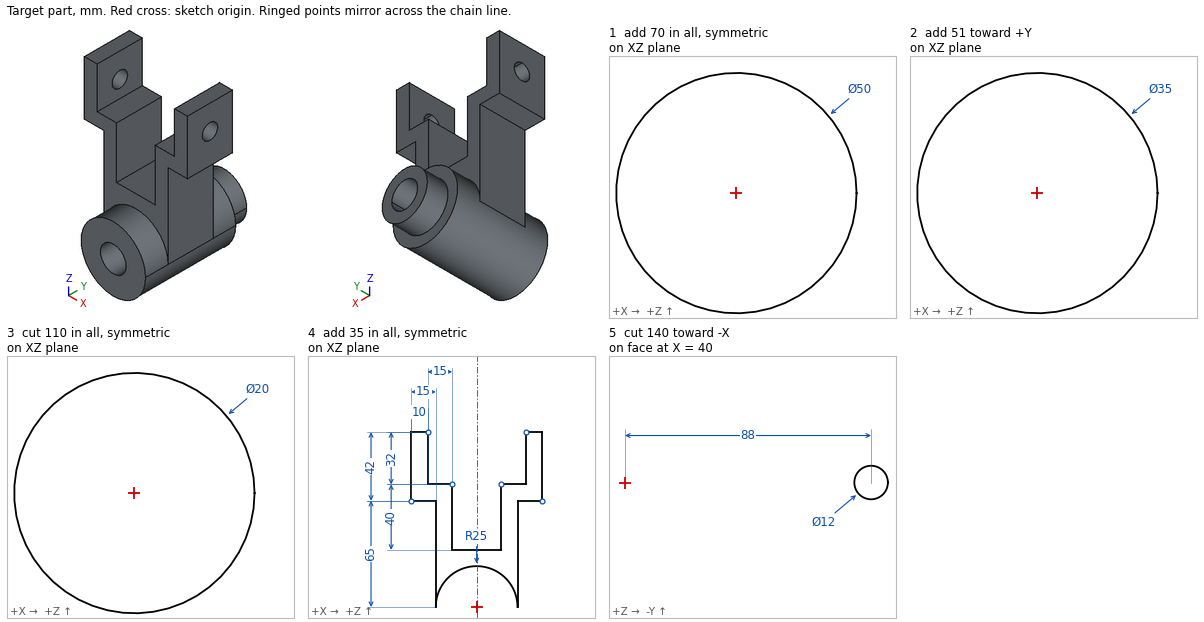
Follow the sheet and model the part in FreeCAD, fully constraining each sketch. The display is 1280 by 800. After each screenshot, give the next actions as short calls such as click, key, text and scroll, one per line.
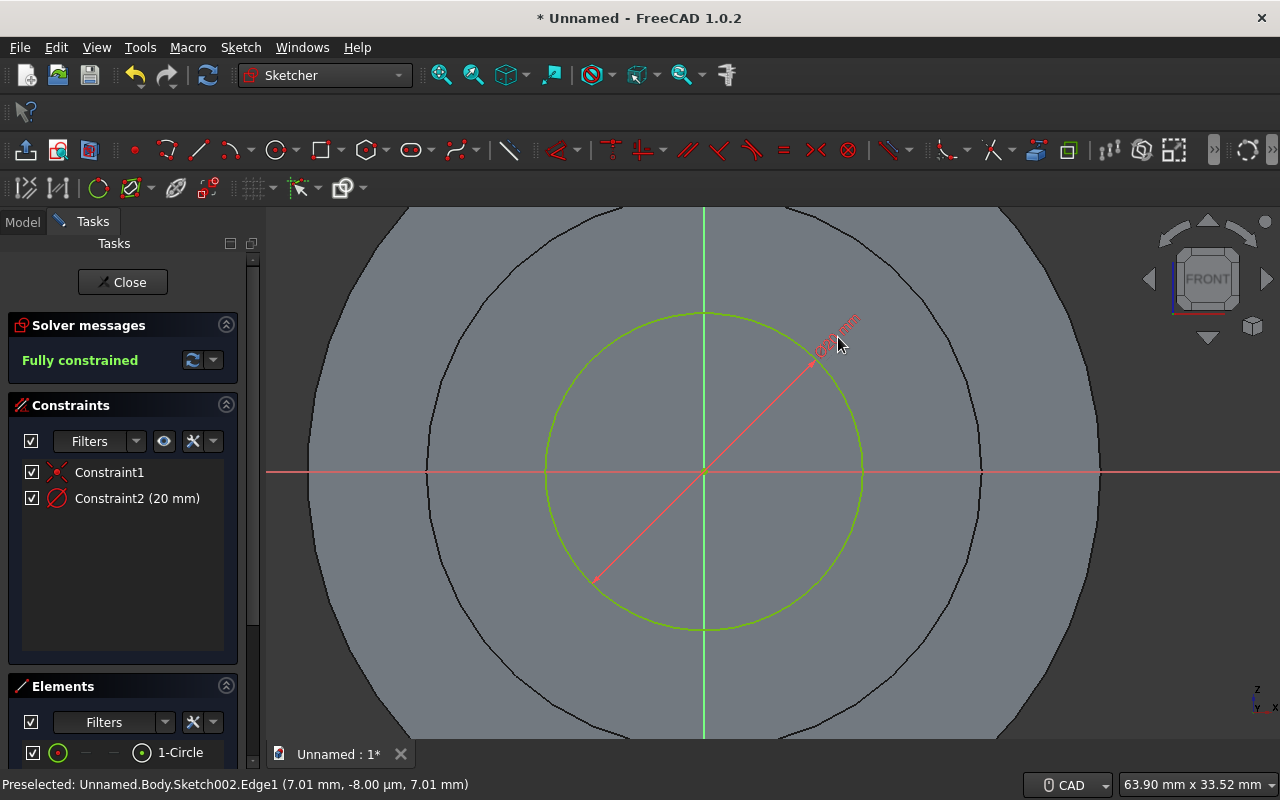
click(123, 282)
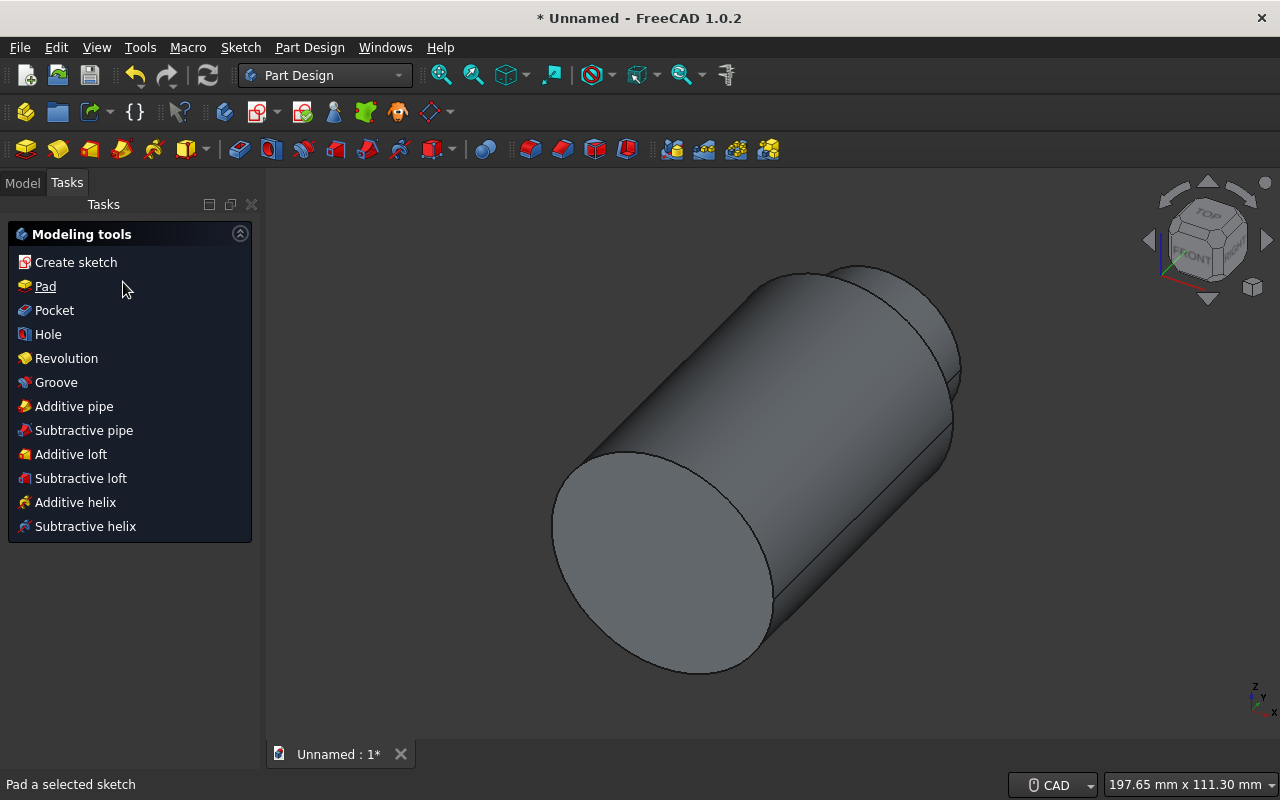
click(240, 150)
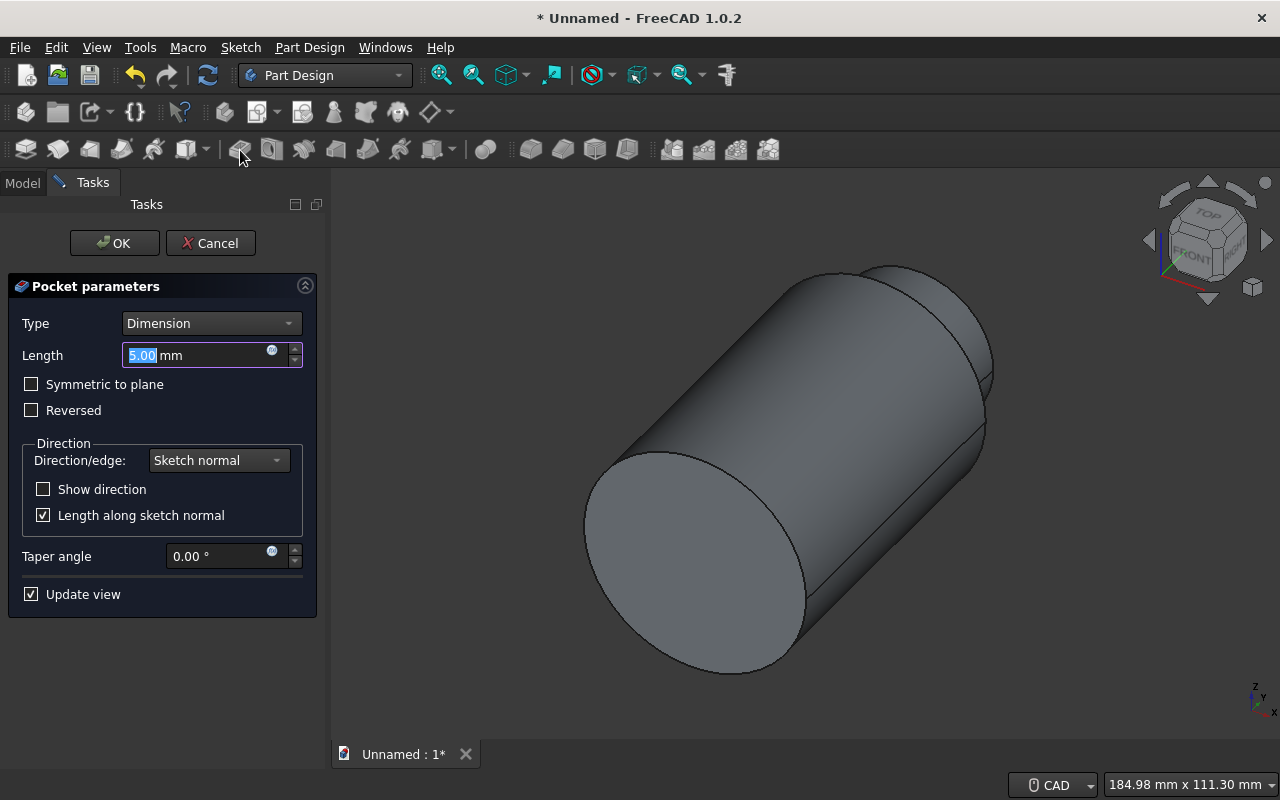
text(110)
key(Tab)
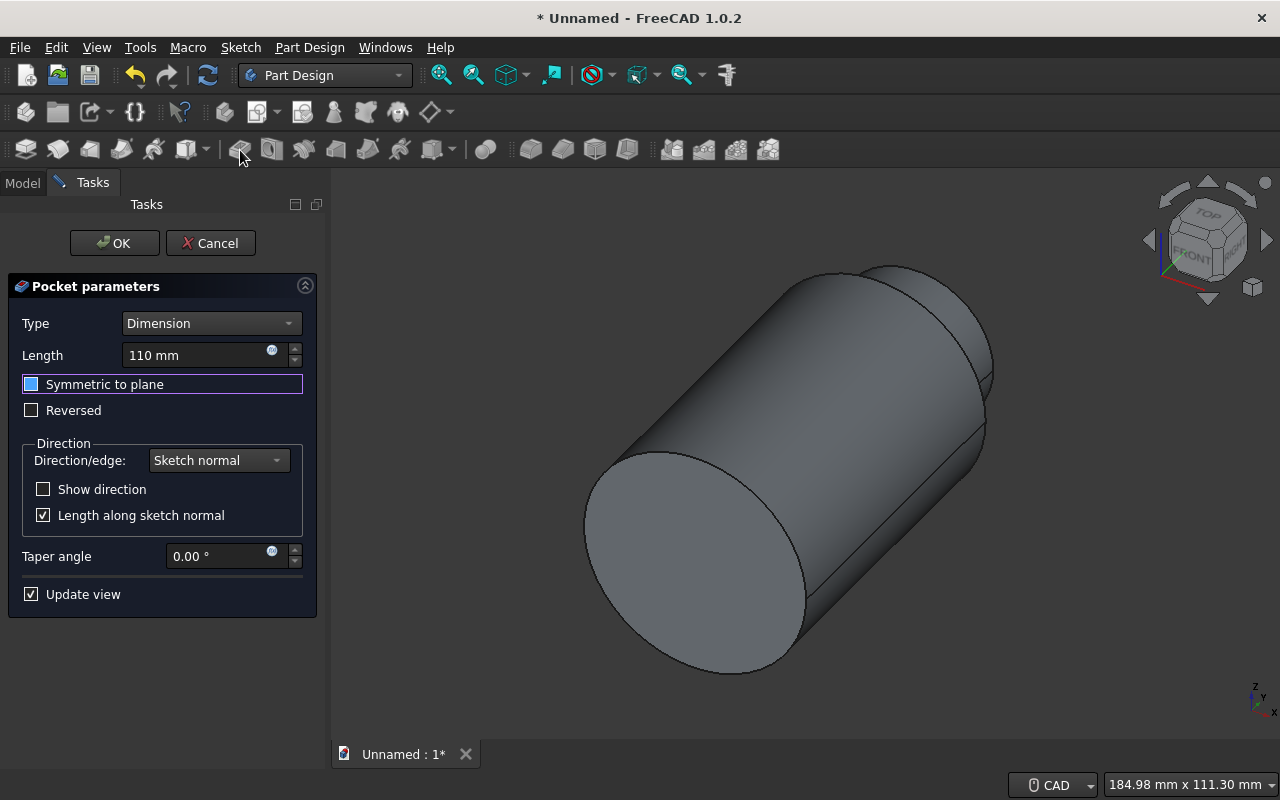
click(30, 384)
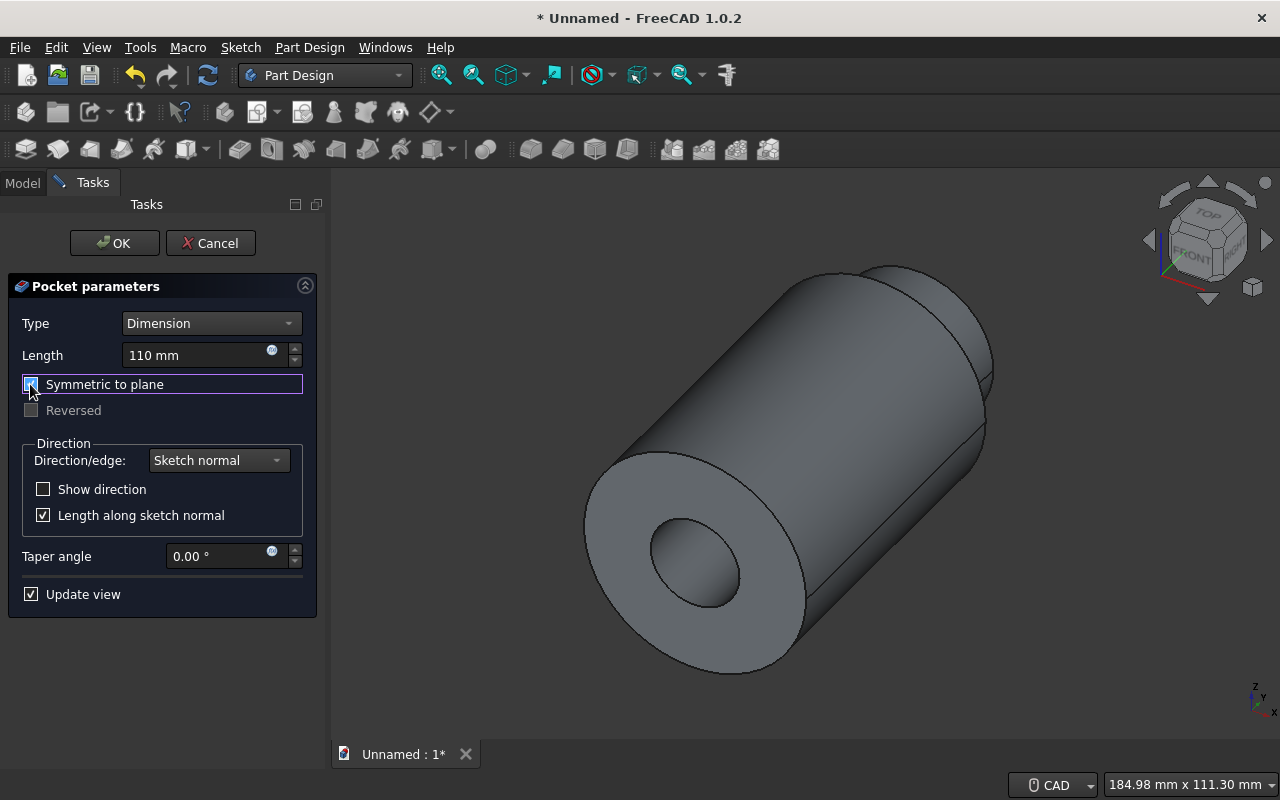
click(115, 243)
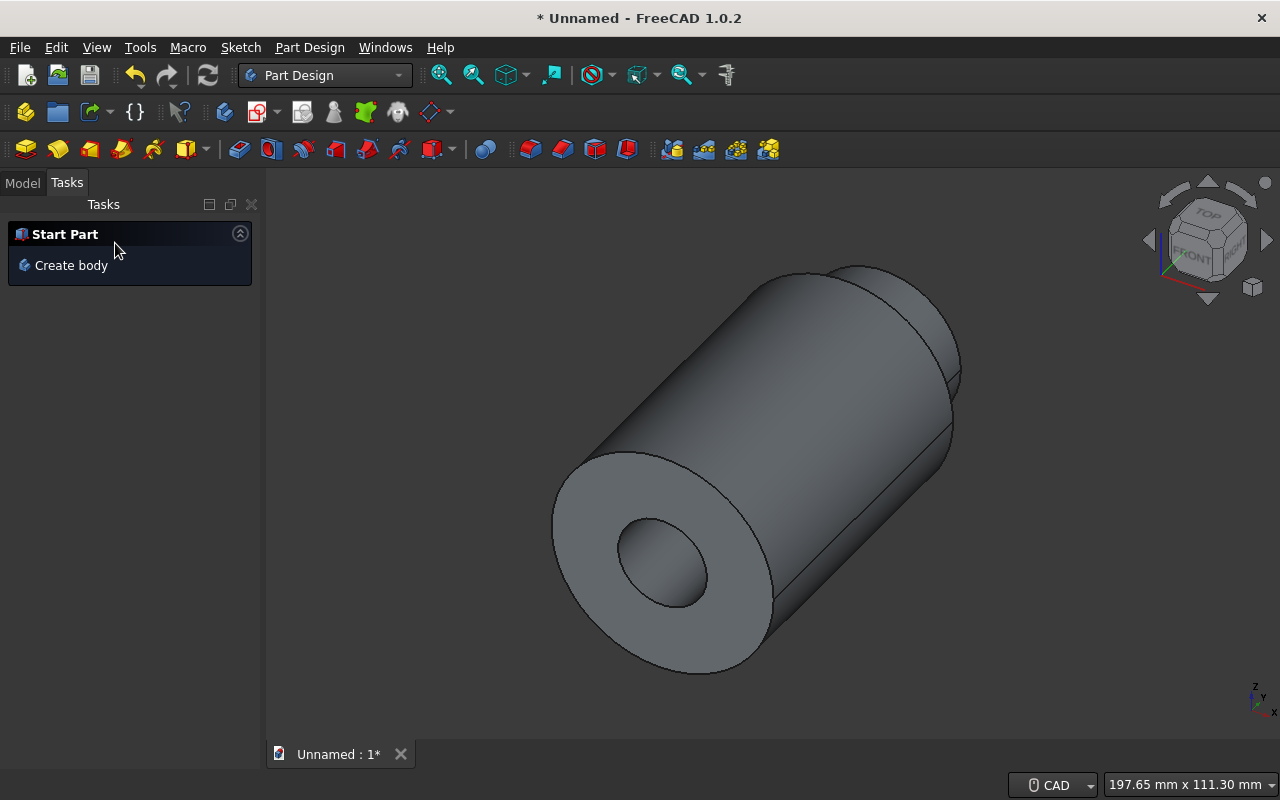
click(258, 112)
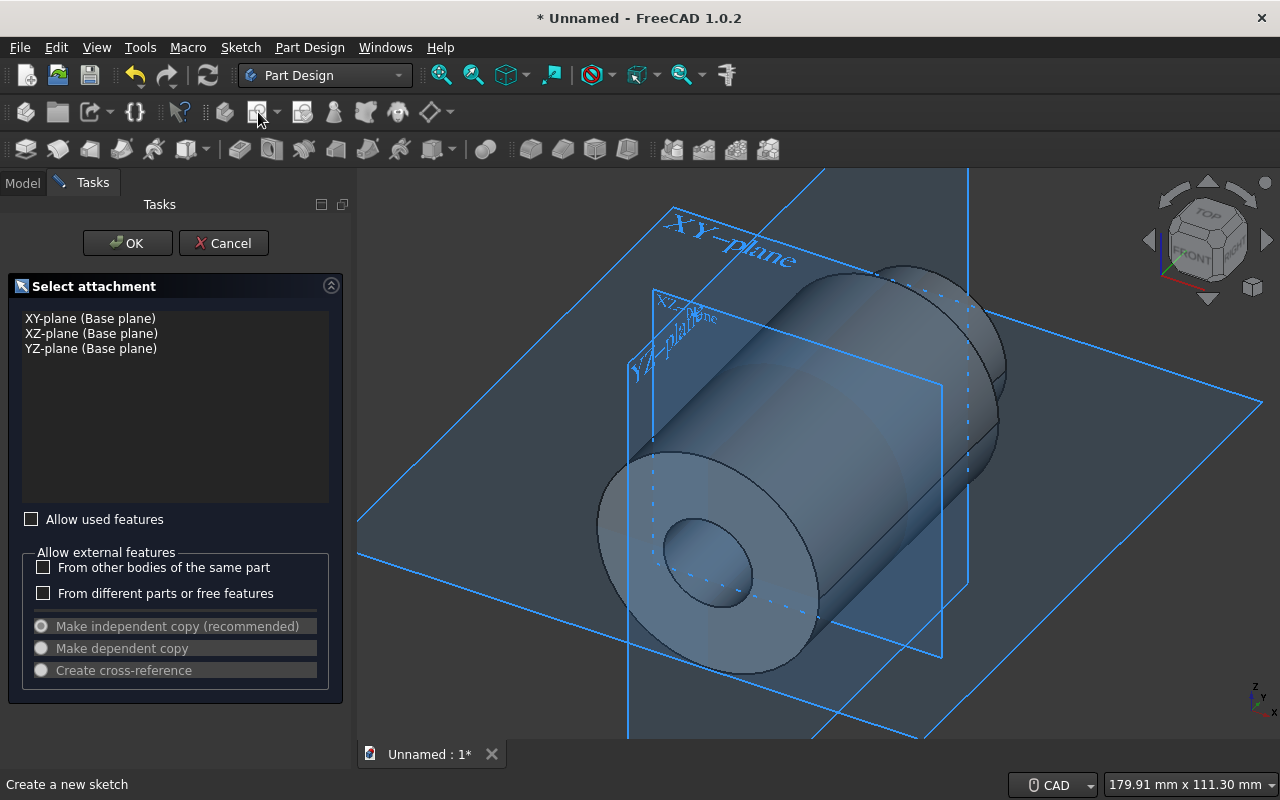
click(82, 334)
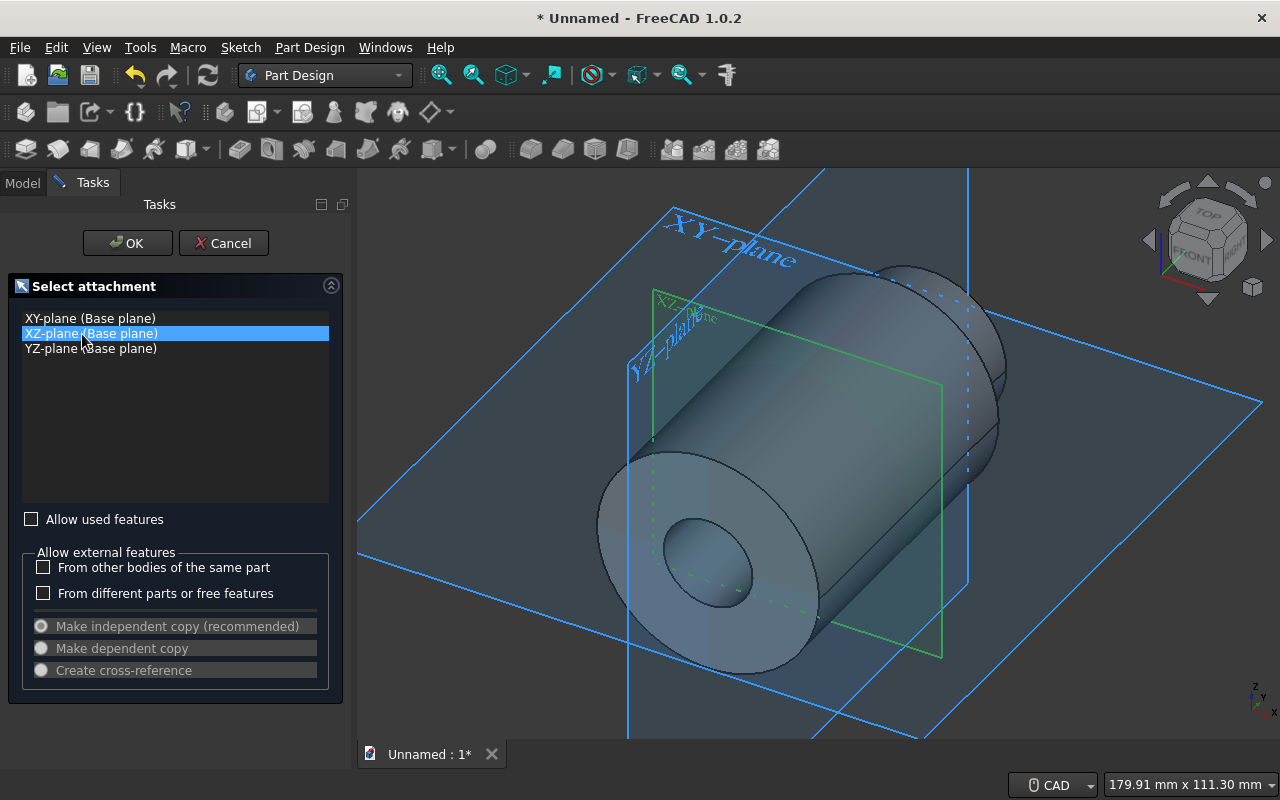
click(128, 243)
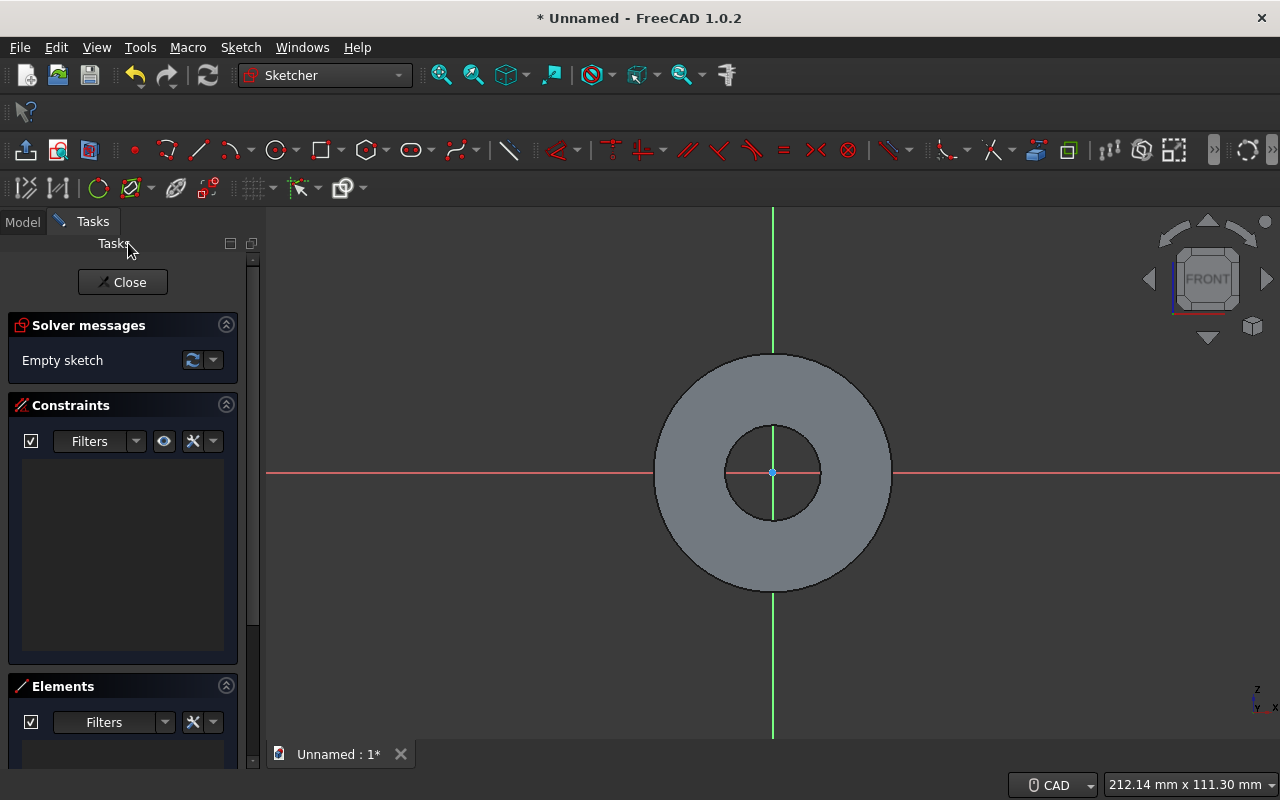
click(90, 150)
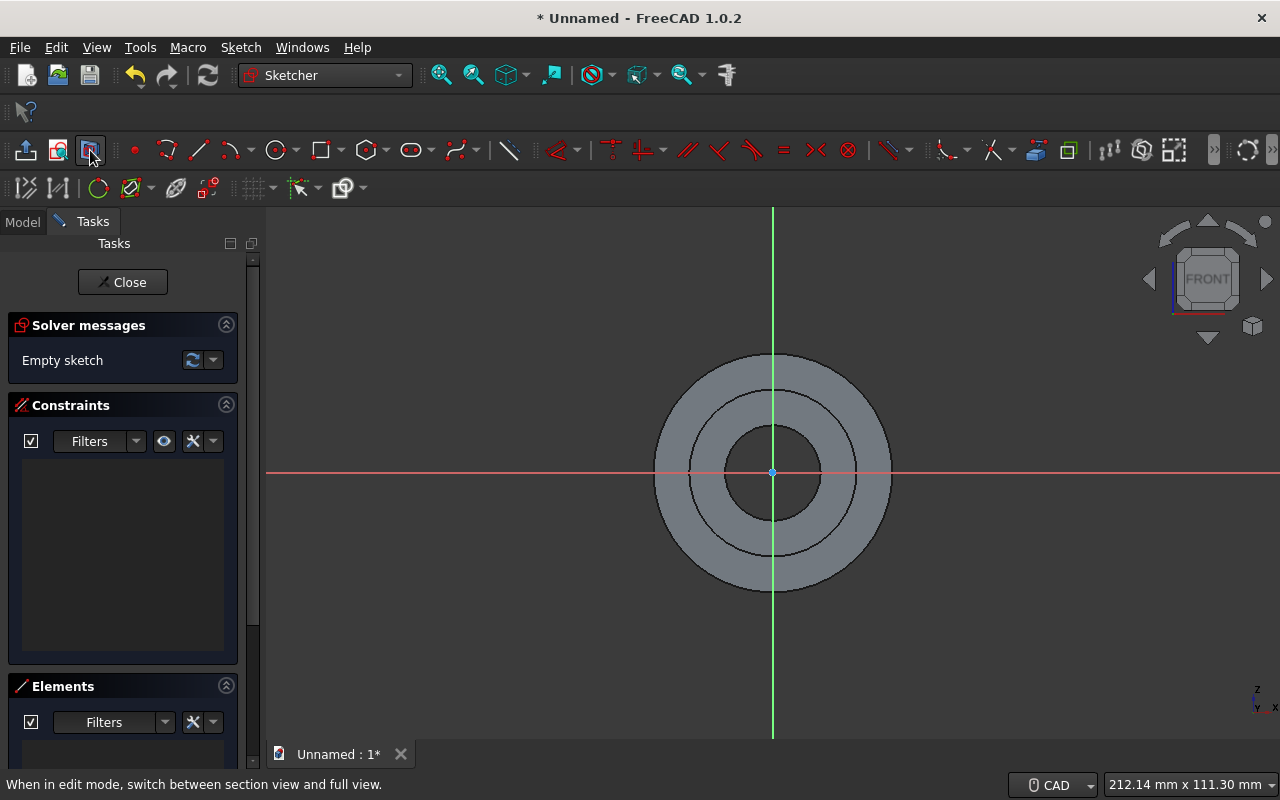
scroll(621, 711, down, 3)